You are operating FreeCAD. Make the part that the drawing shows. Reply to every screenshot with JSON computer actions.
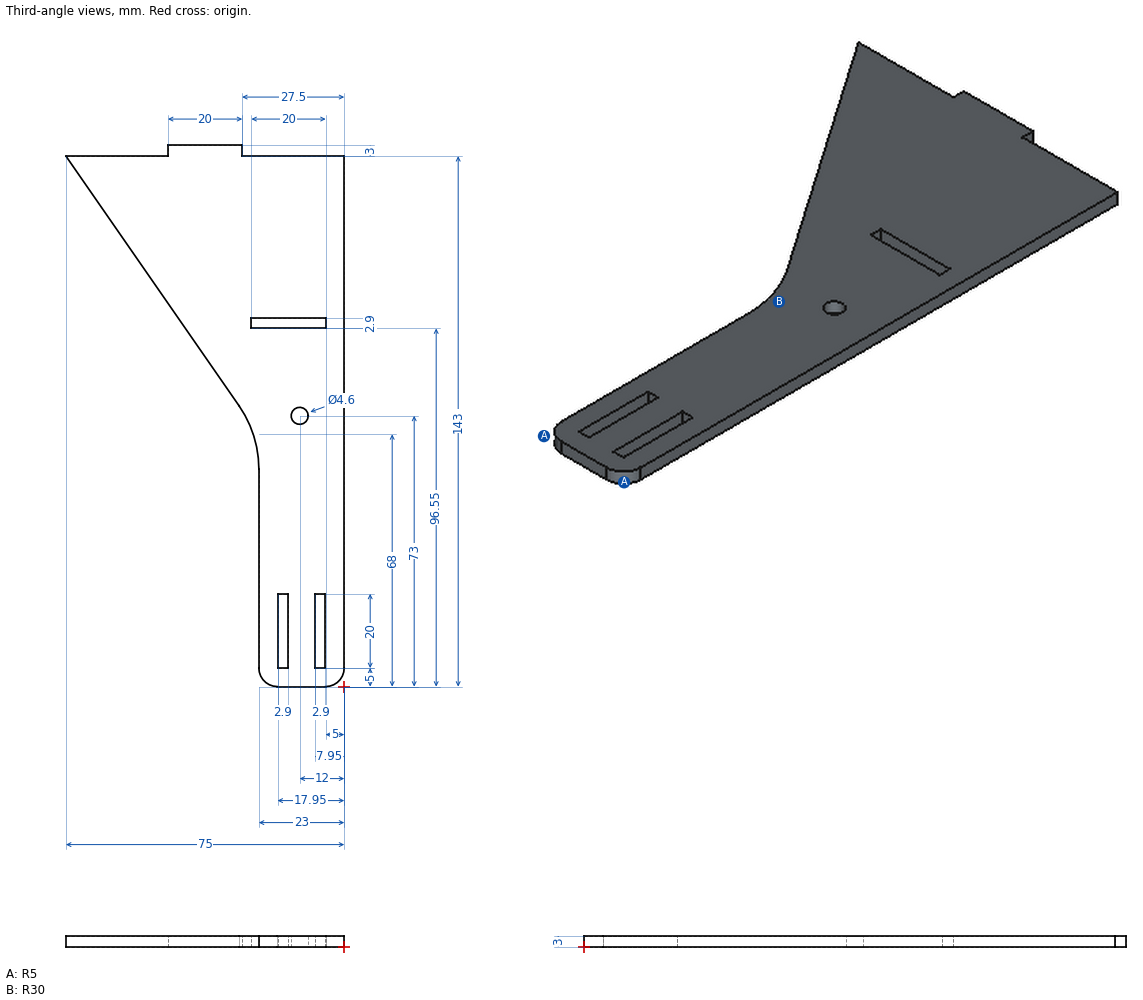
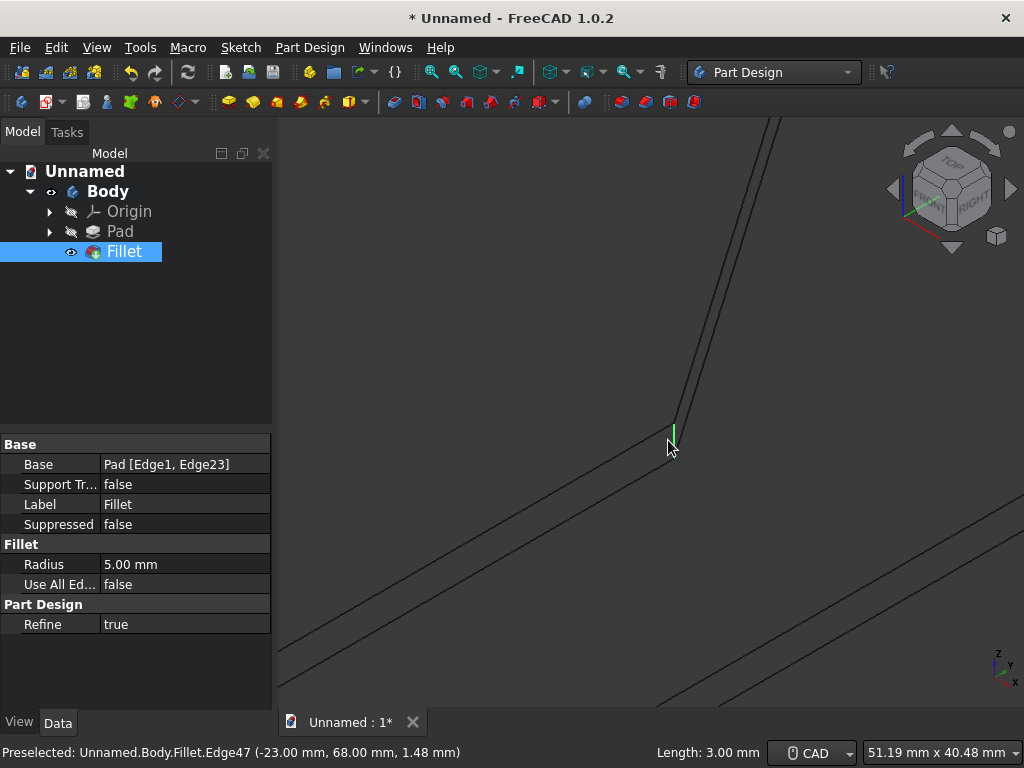
{"action": "key", "text": "v 1"}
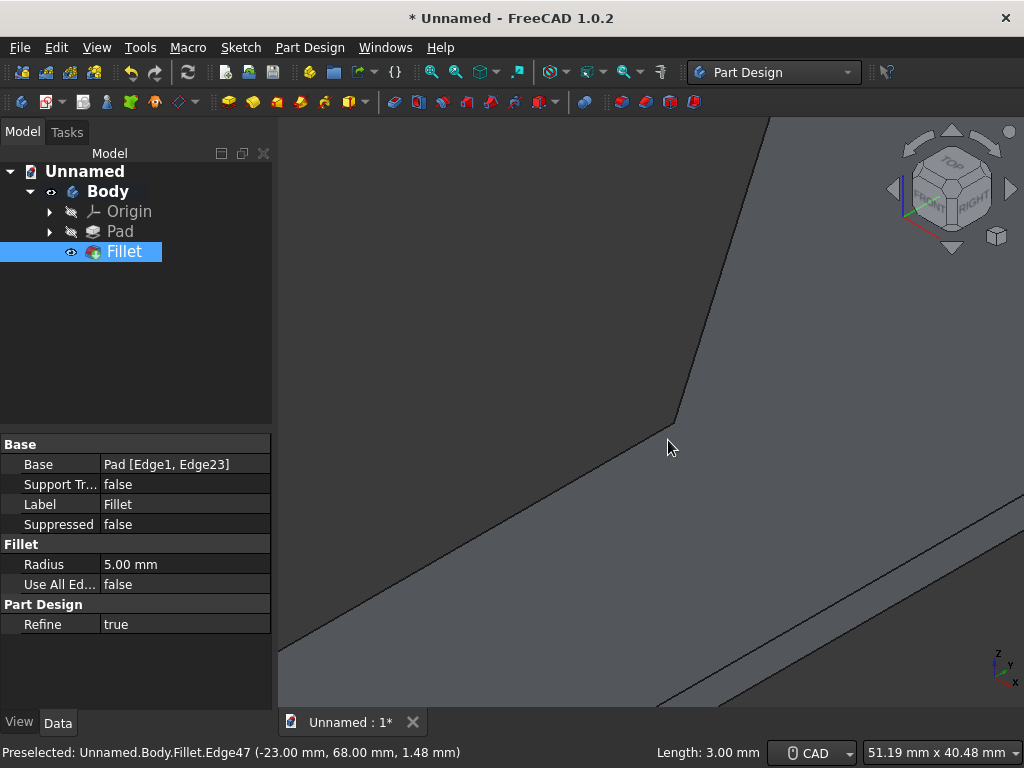
{"action": "left_click", "coordinate": [622, 102]}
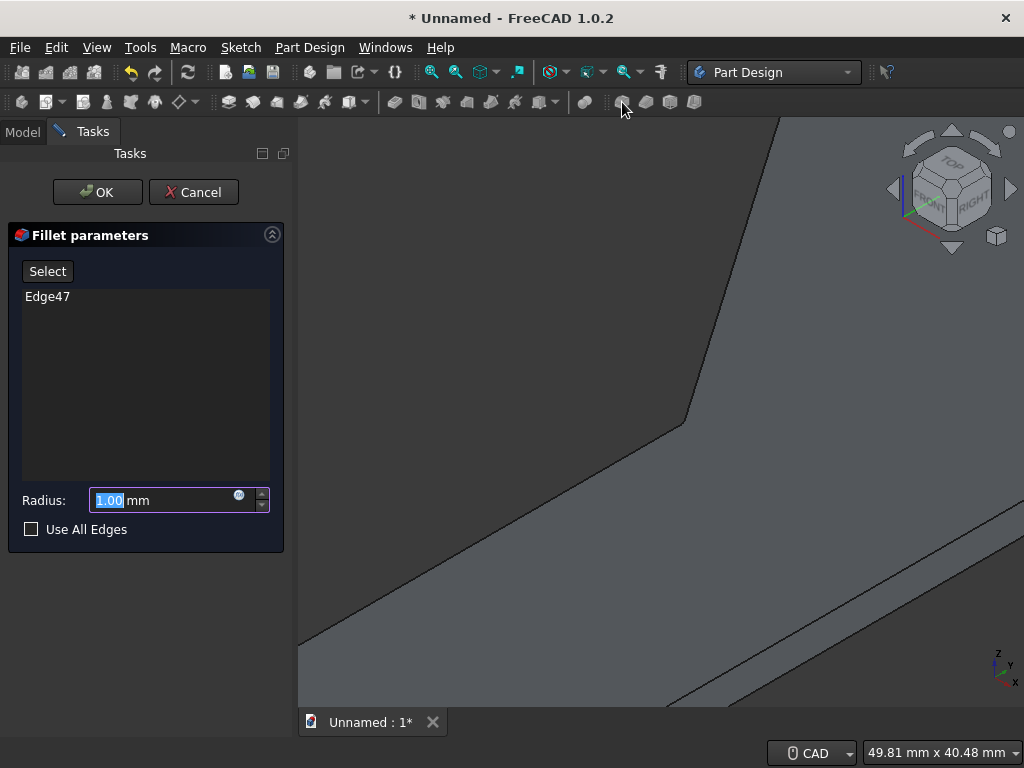
{"action": "type", "text": "30"}
{"action": "key", "text": "Tab"}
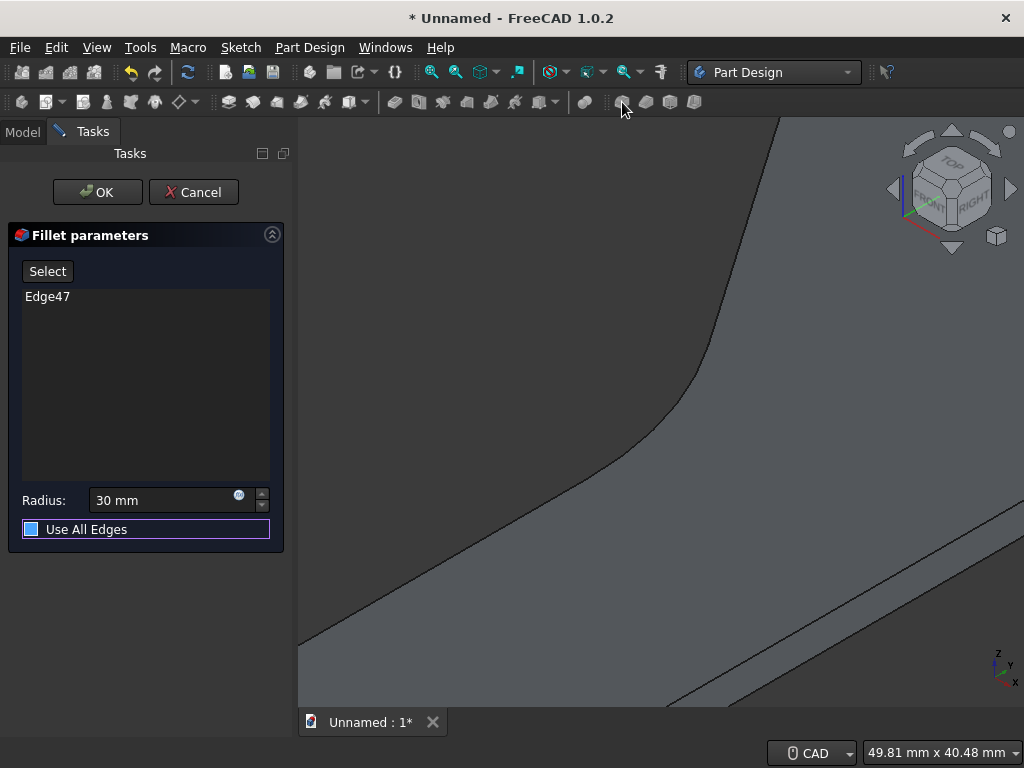
{"action": "left_click", "coordinate": [98, 192]}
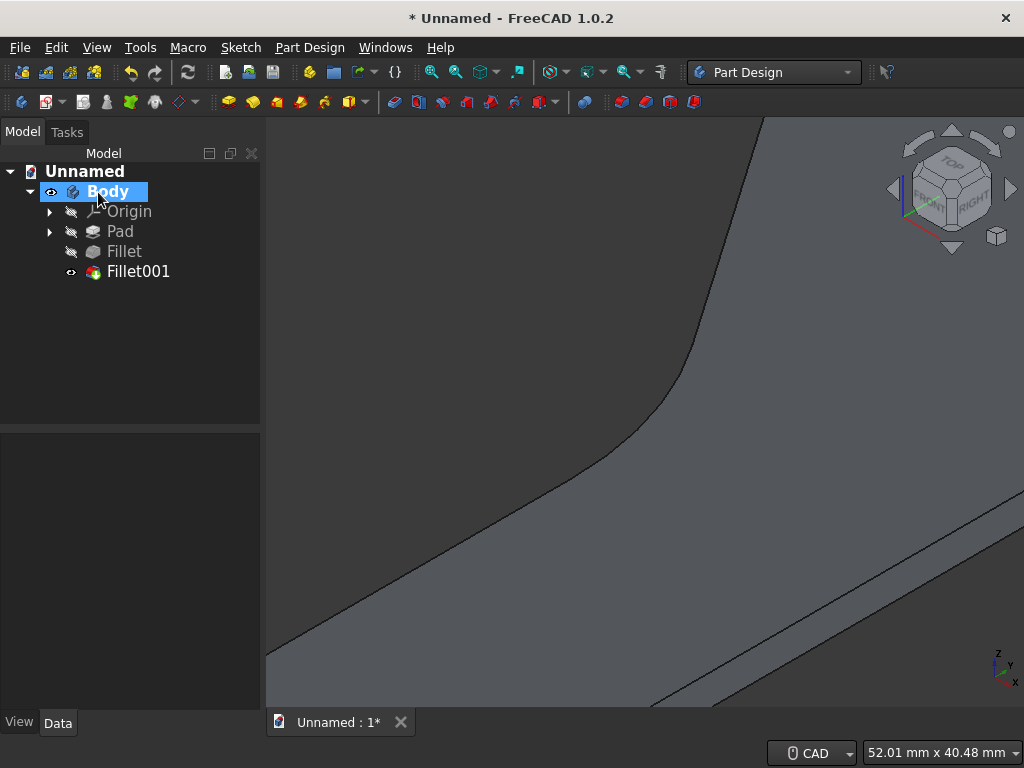
{"action": "key", "text": "v f"}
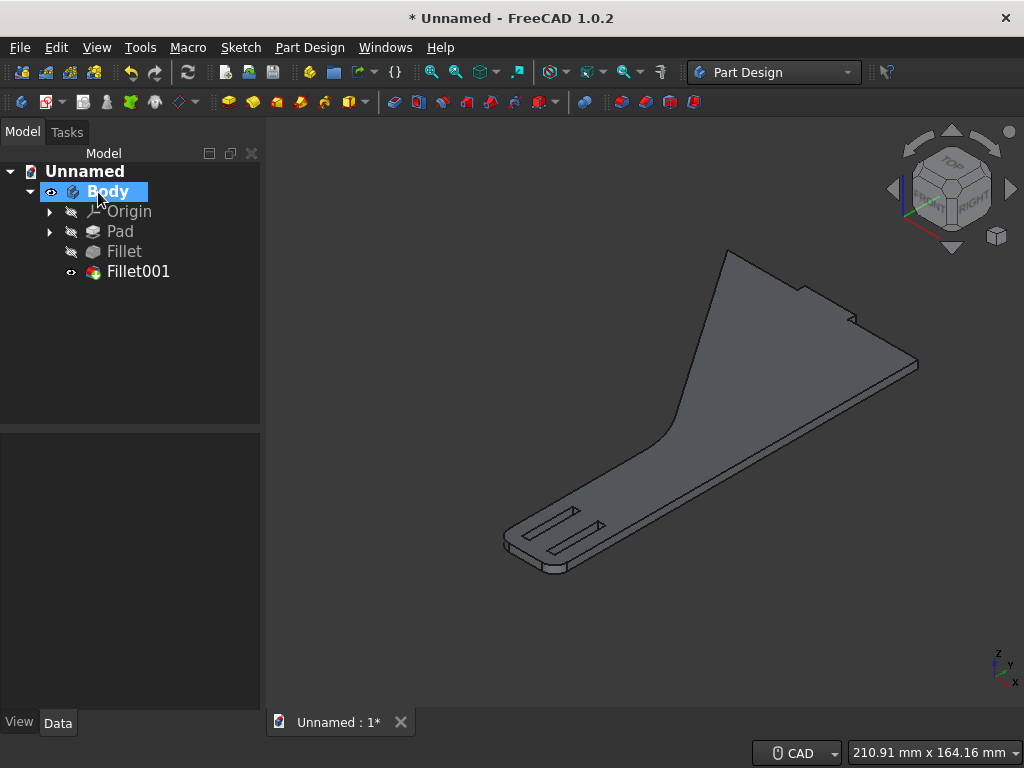
{"action": "left_click", "coordinate": [778, 361]}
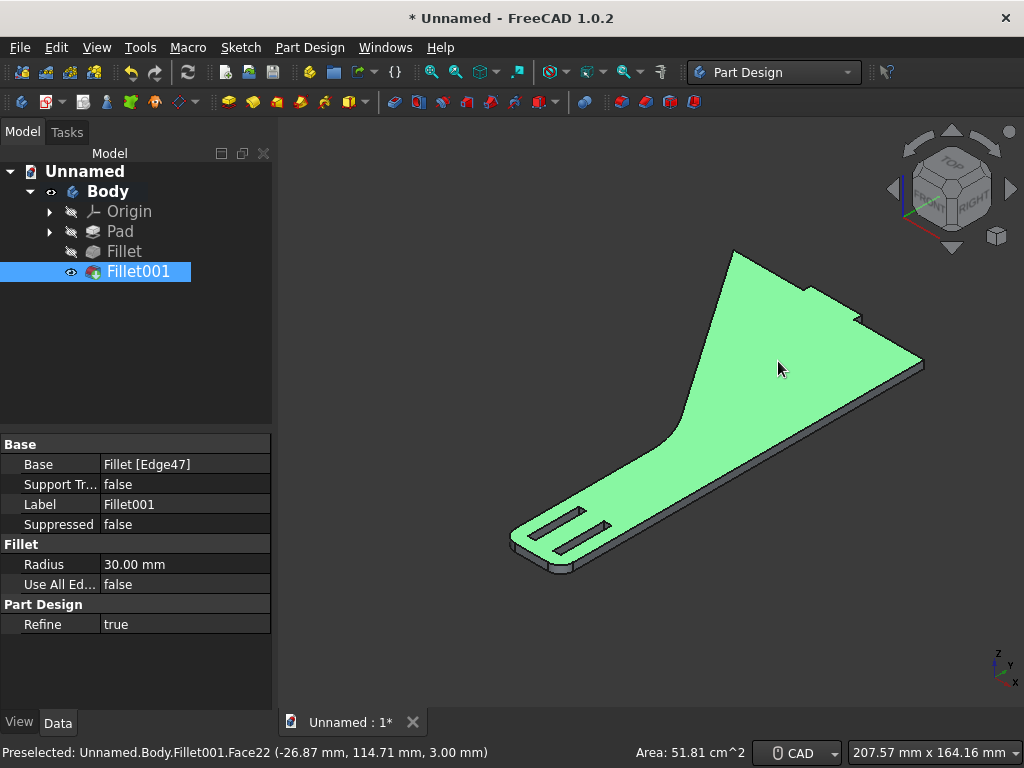
{"action": "left_click", "coordinate": [46, 102]}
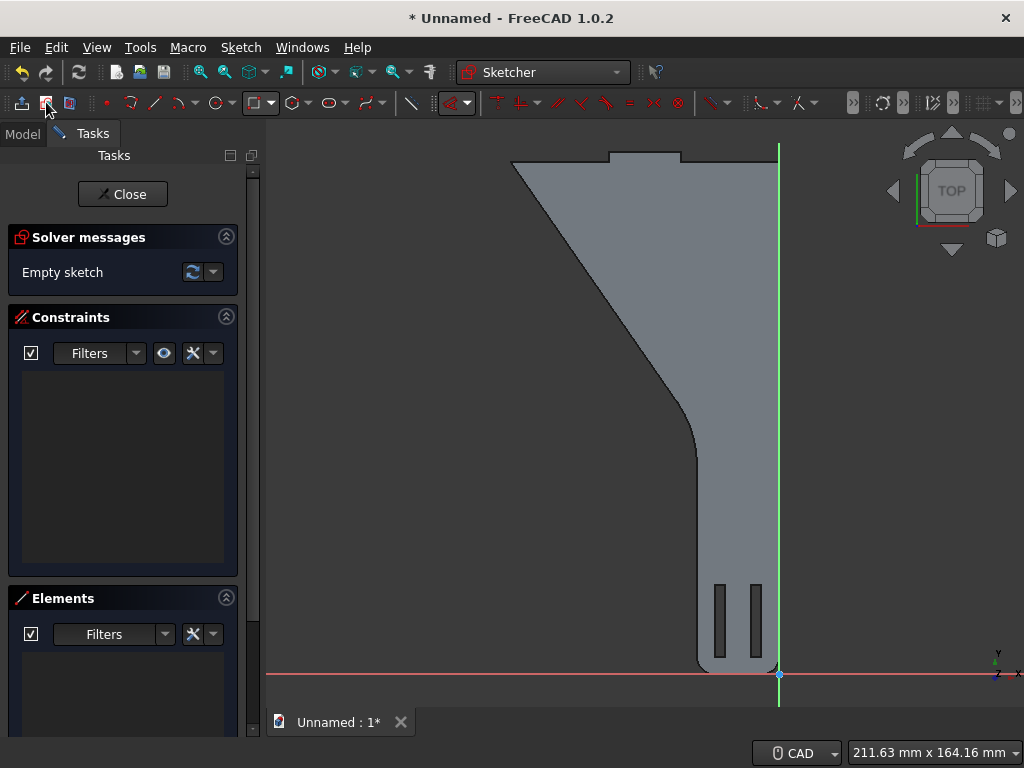
{"action": "scroll", "coordinate": [745, 413], "scroll_direction": "up", "scroll_amount": 15}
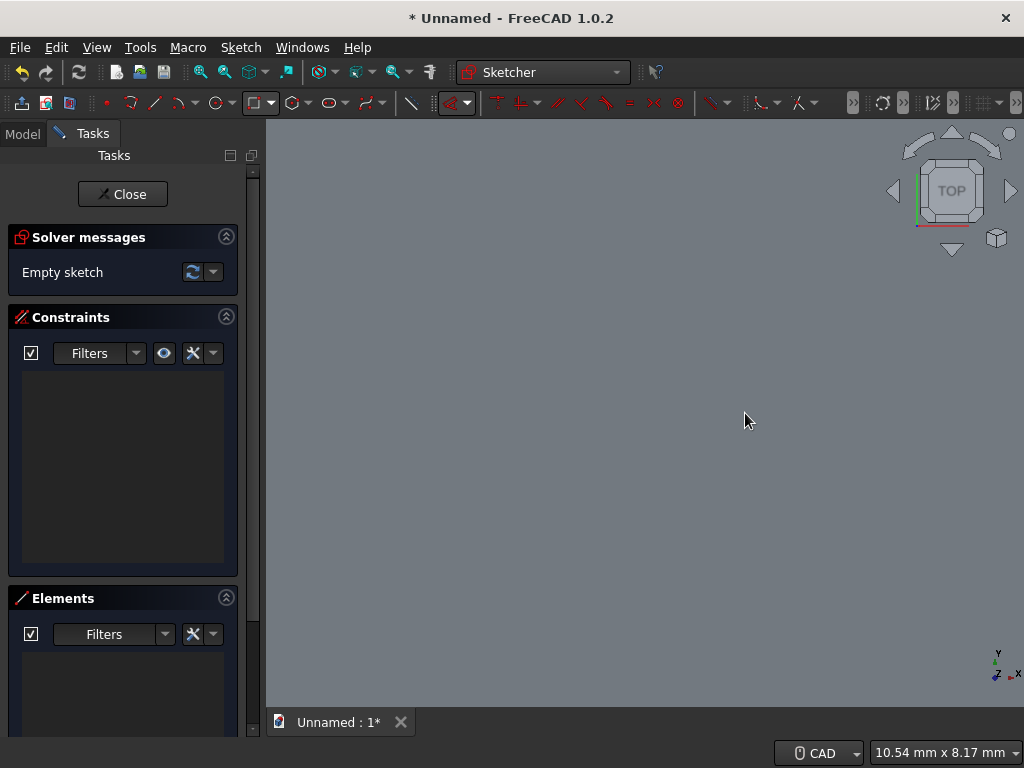
{"action": "left_click", "coordinate": [216, 104]}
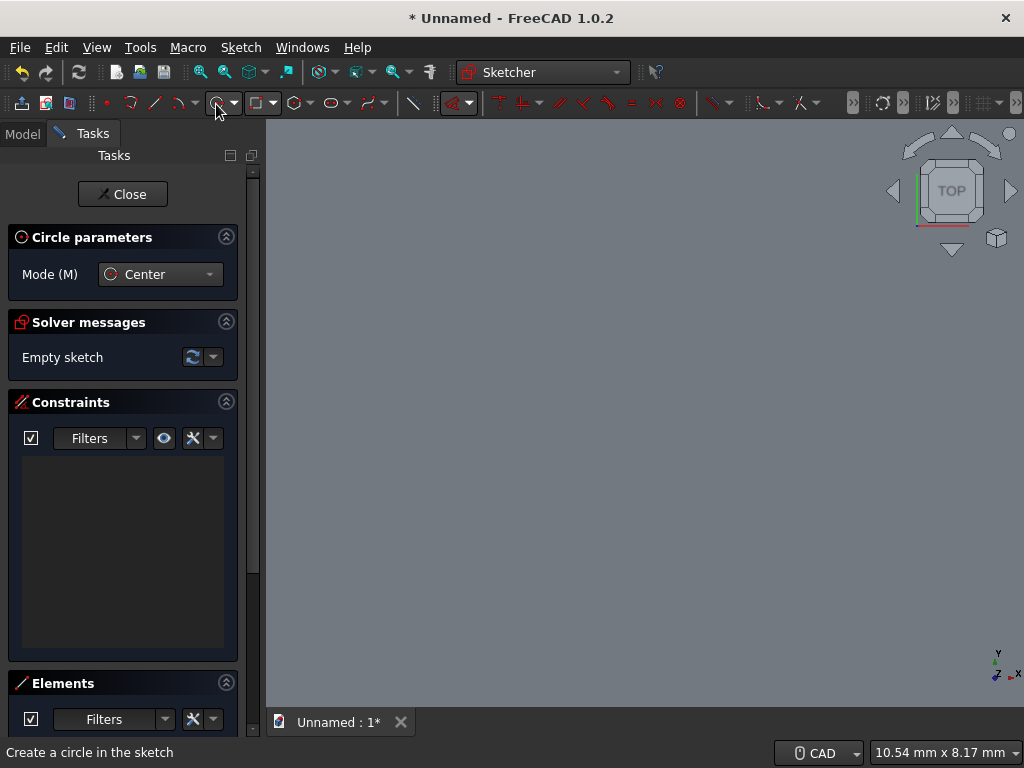
{"action": "left_click", "coordinate": [559, 403]}
{"action": "mouse_move", "coordinate": [676, 286]}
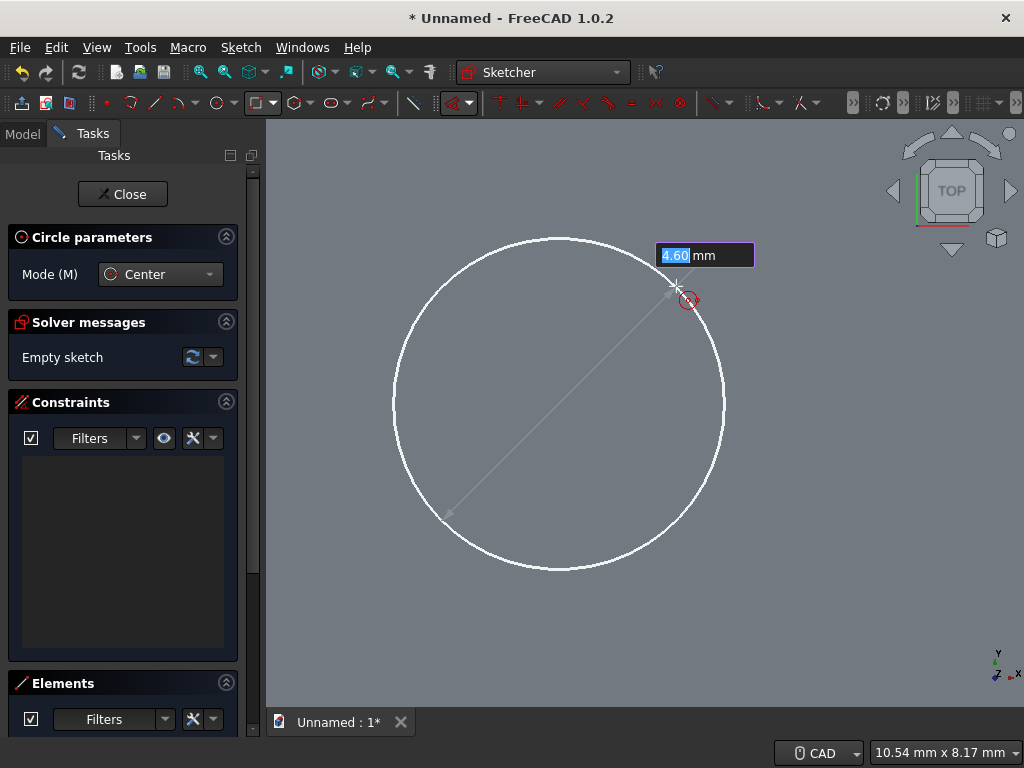
{"action": "type", "text": "4.6"}
{"action": "key", "text": "Return"}
{"action": "key", "text": "Escape"}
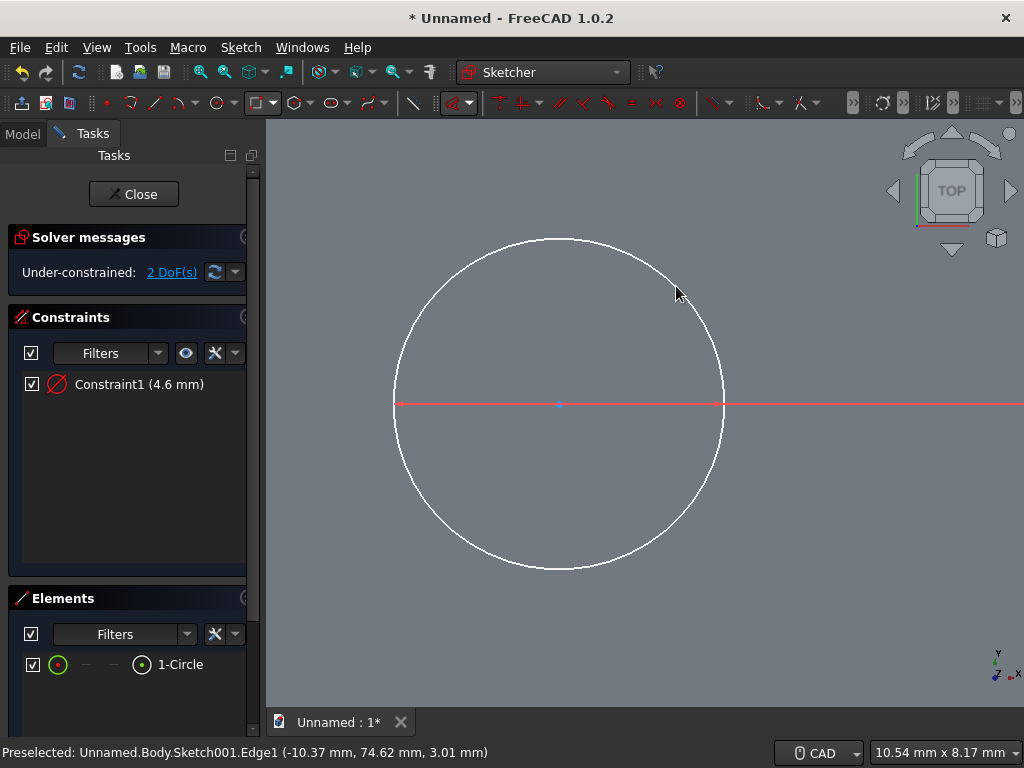
{"action": "left_click", "coordinate": [559, 404]}